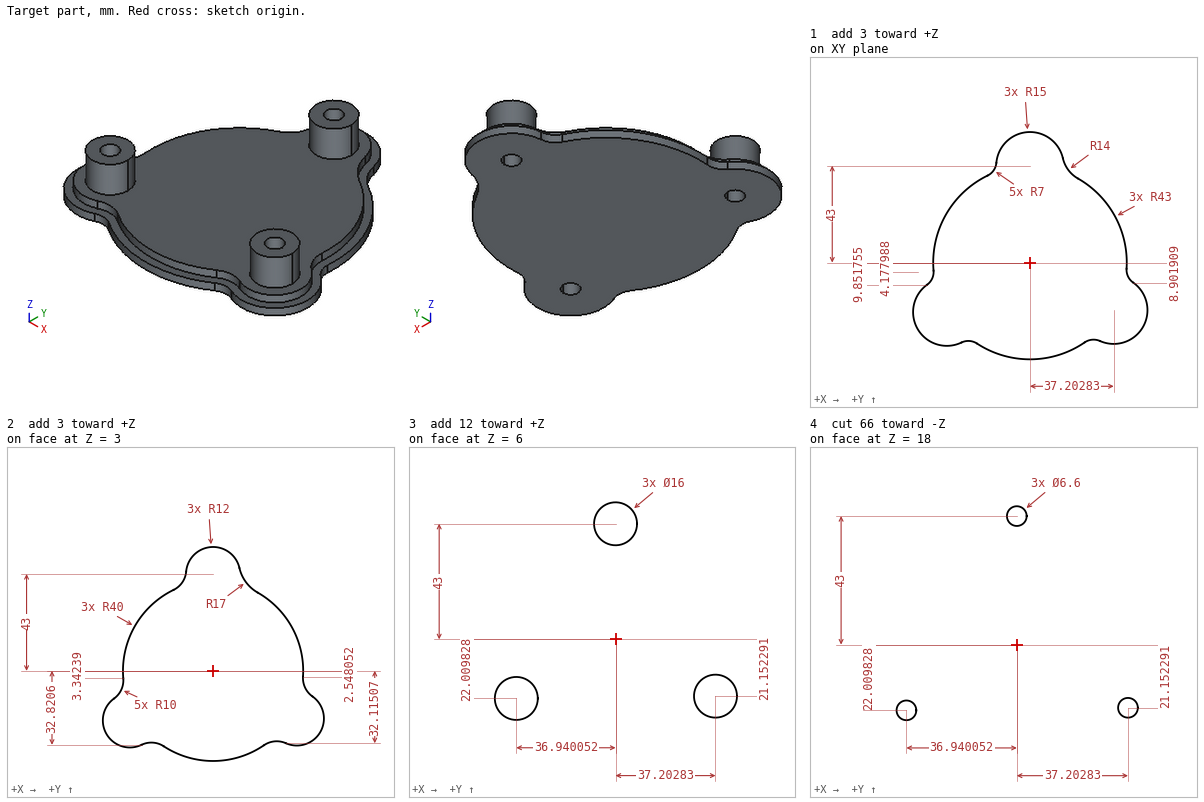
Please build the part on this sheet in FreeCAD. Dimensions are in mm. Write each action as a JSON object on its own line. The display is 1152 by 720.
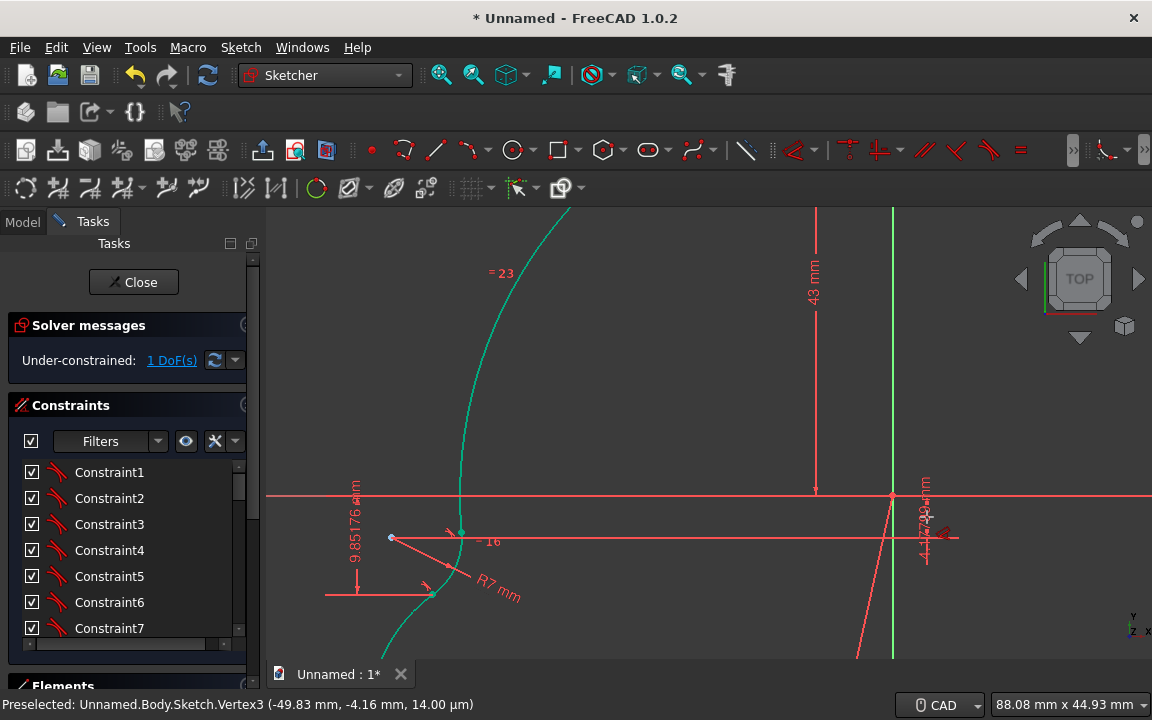
{"action": "scroll", "coordinate": [531, 438], "scroll_direction": "down", "scroll_amount": 6}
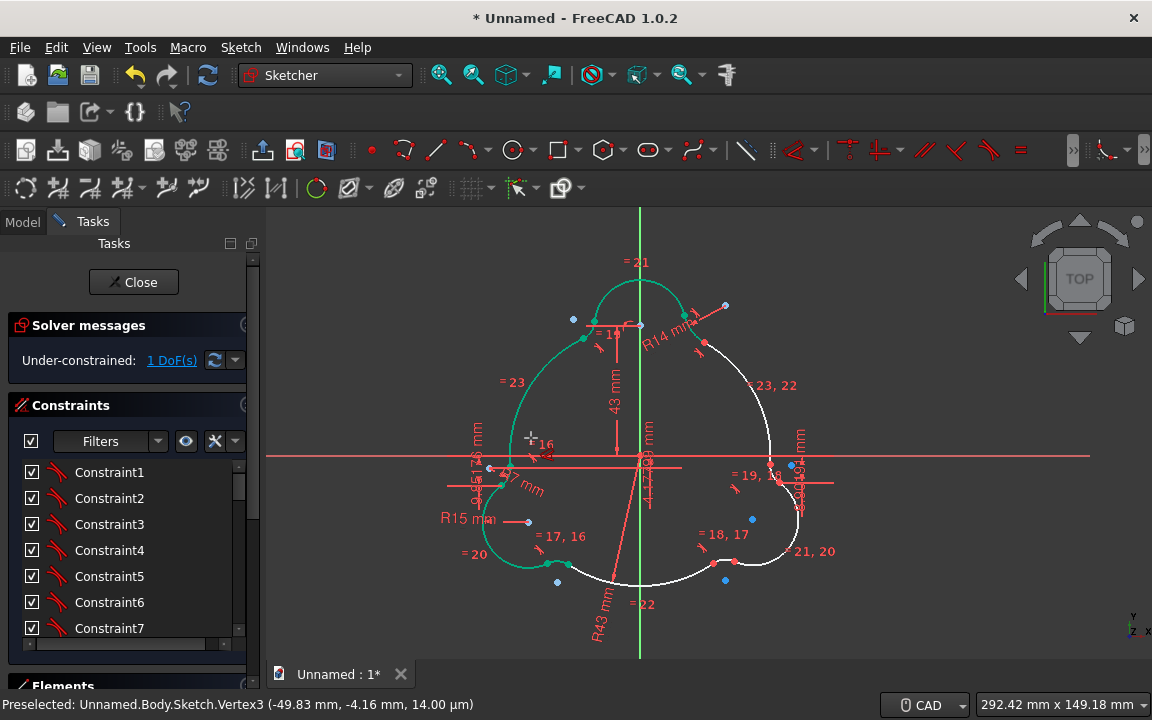
{"action": "left_click", "coordinate": [753, 520]}
{"action": "left_click", "coordinate": [697, 554]}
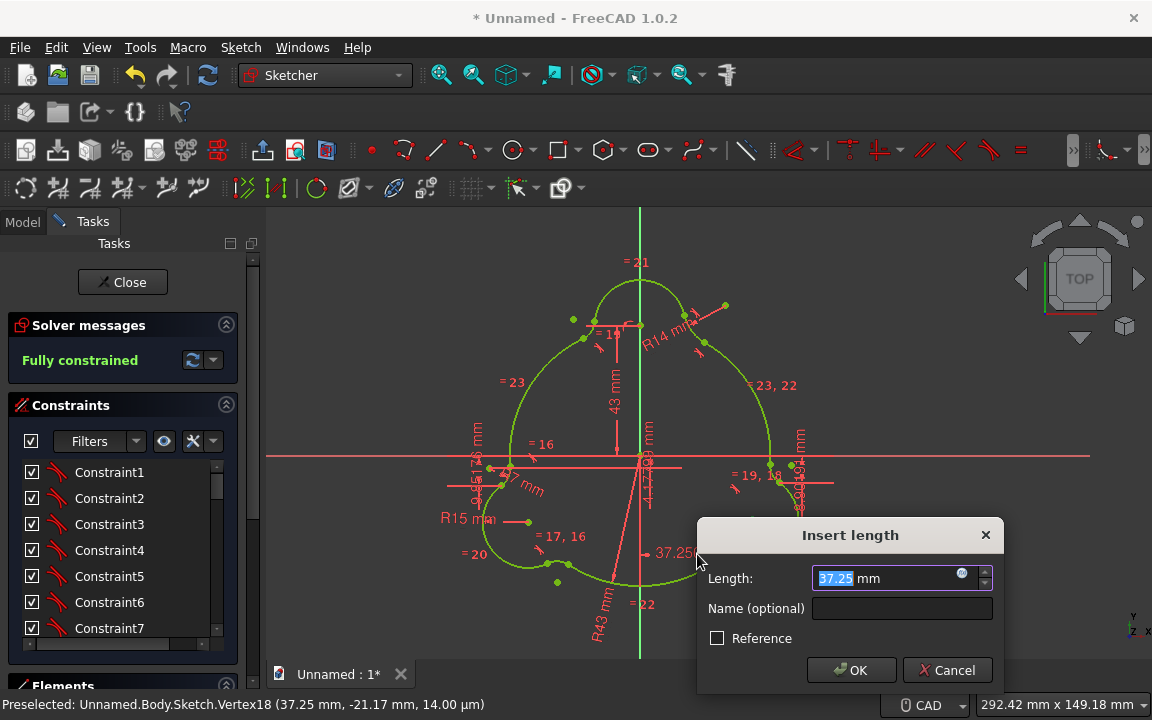
{"action": "type", "text": "37.20283"}
{"action": "key", "text": "Return"}
{"action": "key", "text": "Escape"}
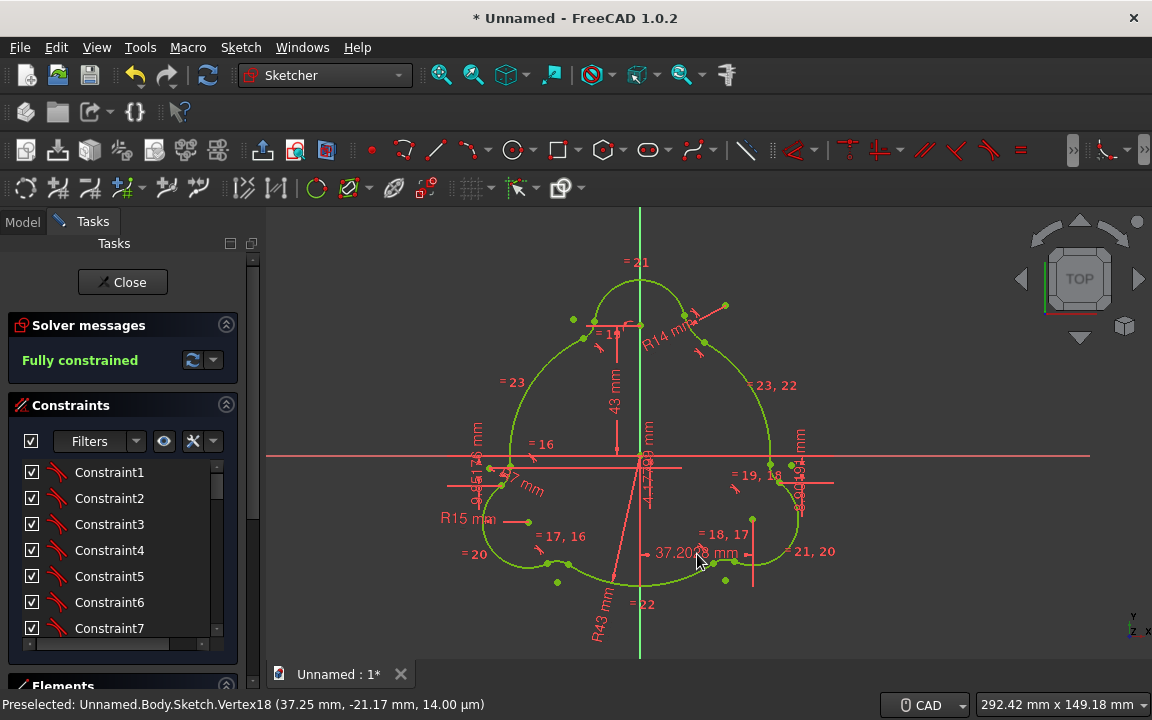
{"action": "left_click", "coordinate": [123, 282]}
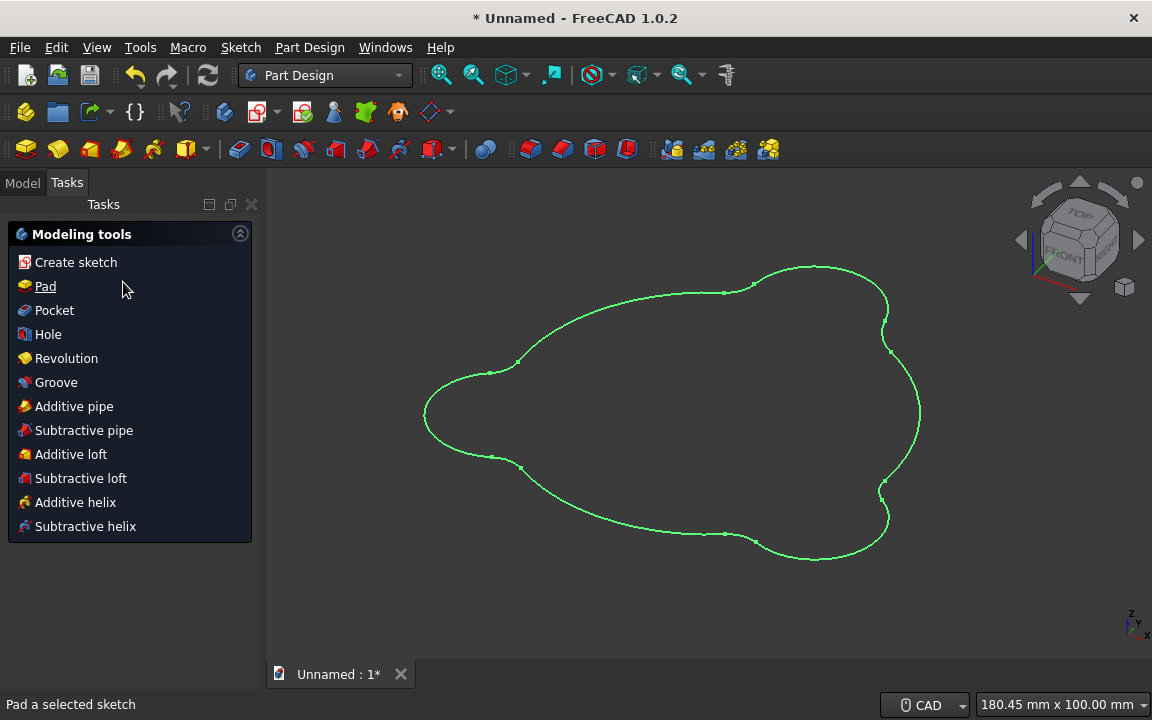
{"action": "left_click", "coordinate": [26, 150]}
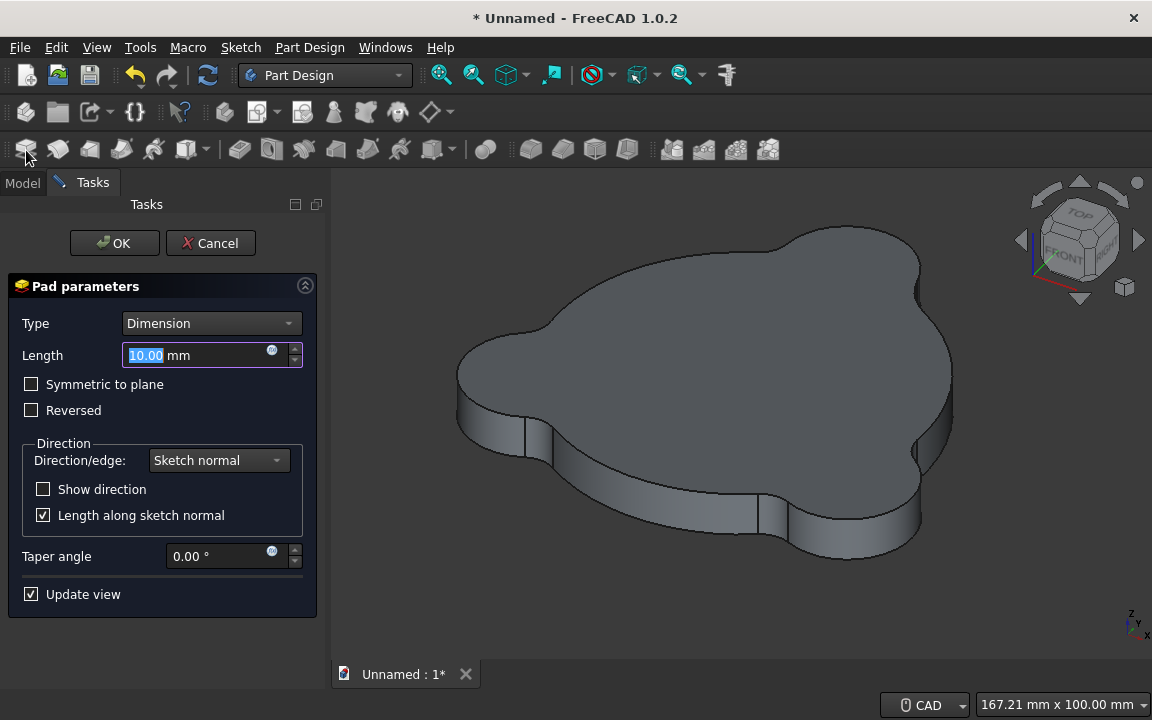
{"action": "type", "text": "3"}
{"action": "key", "text": "Tab"}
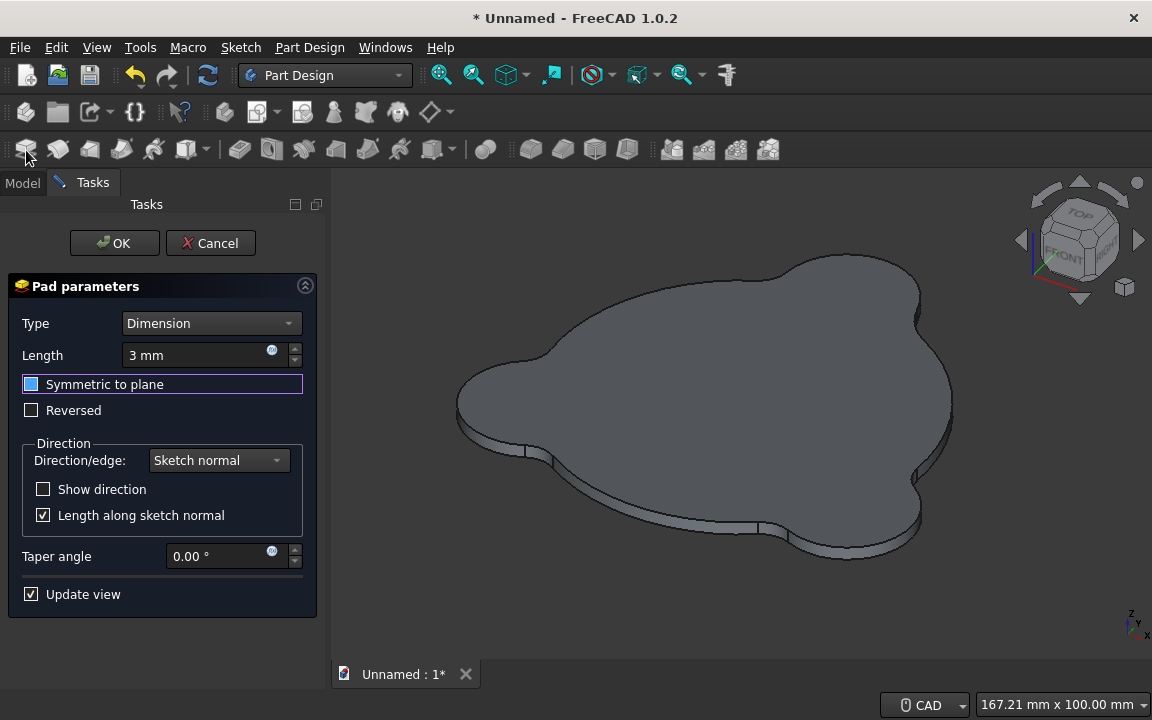
{"action": "left_click", "coordinate": [115, 243]}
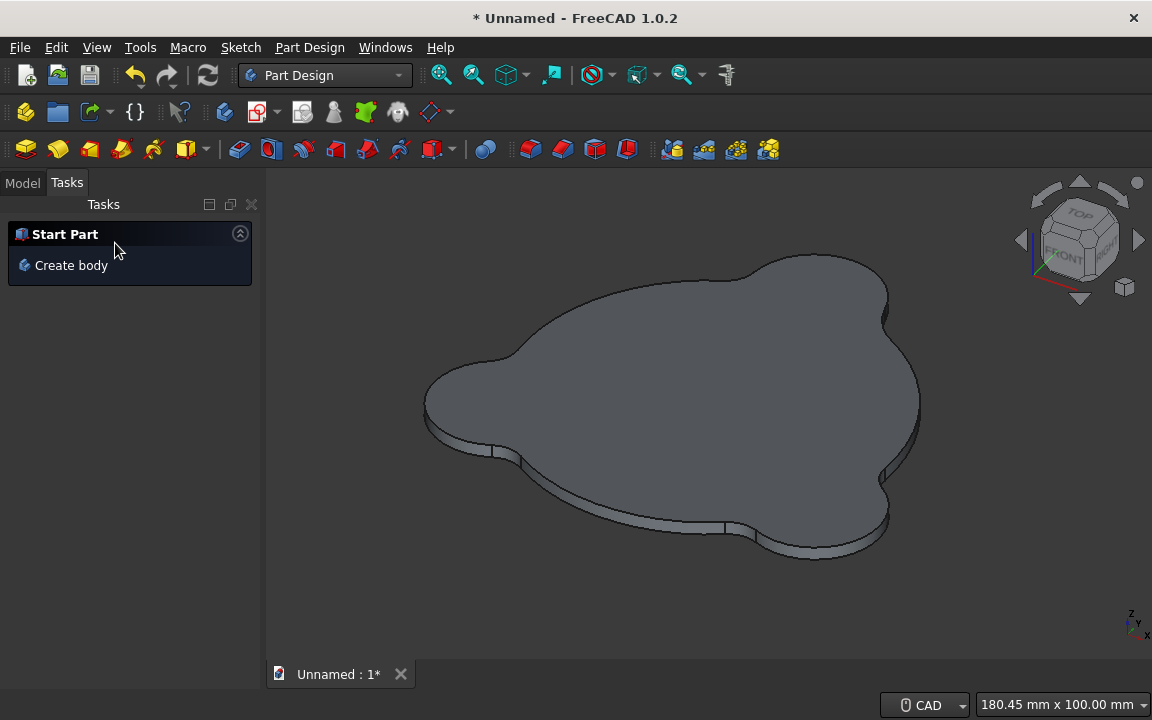
{"action": "left_click", "coordinate": [728, 382]}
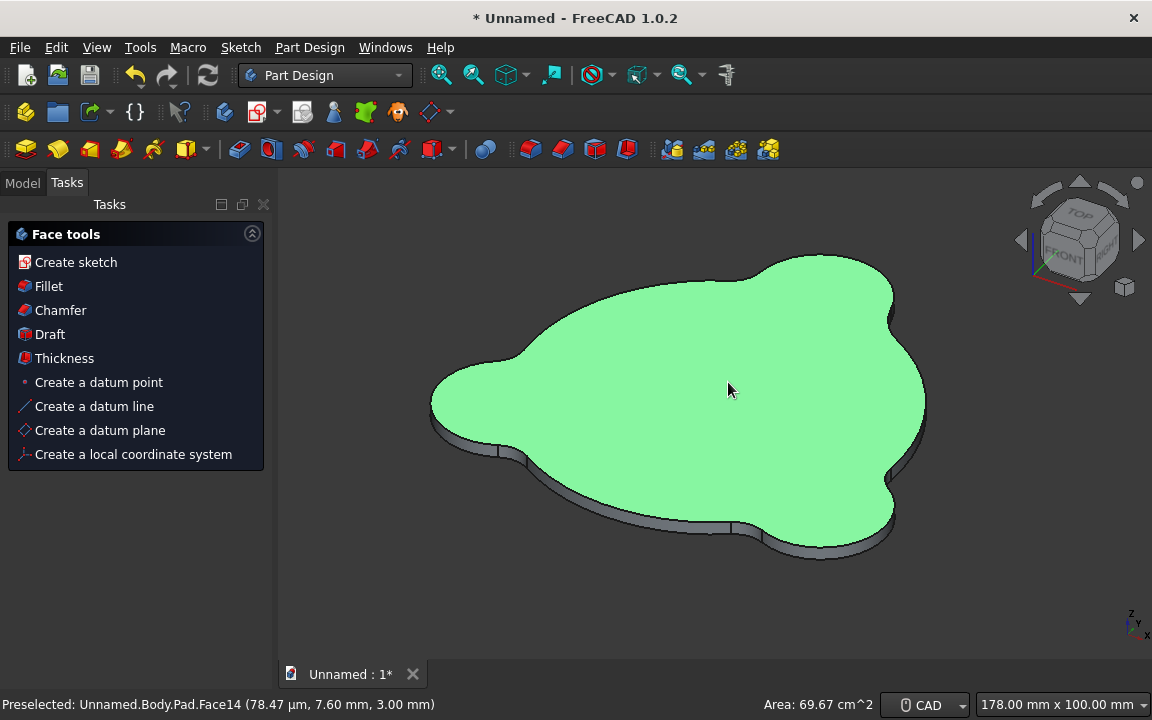
{"action": "left_click", "coordinate": [258, 112]}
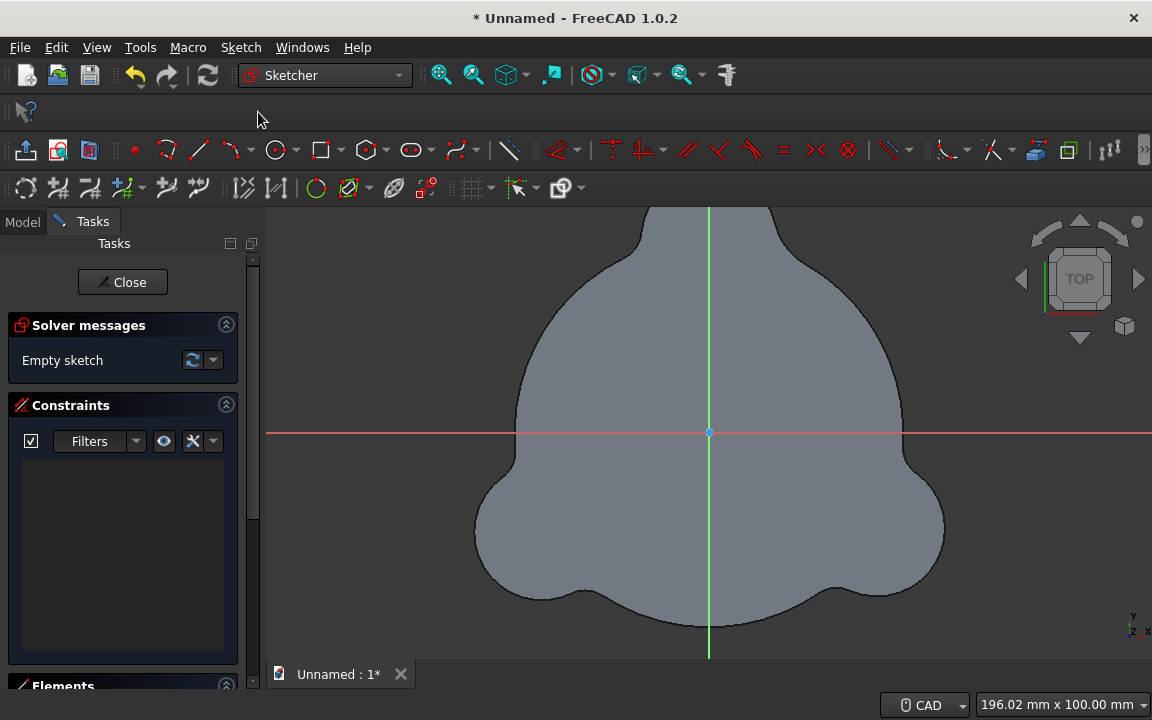
{"action": "scroll", "coordinate": [499, 502], "scroll_direction": "down", "scroll_amount": 2}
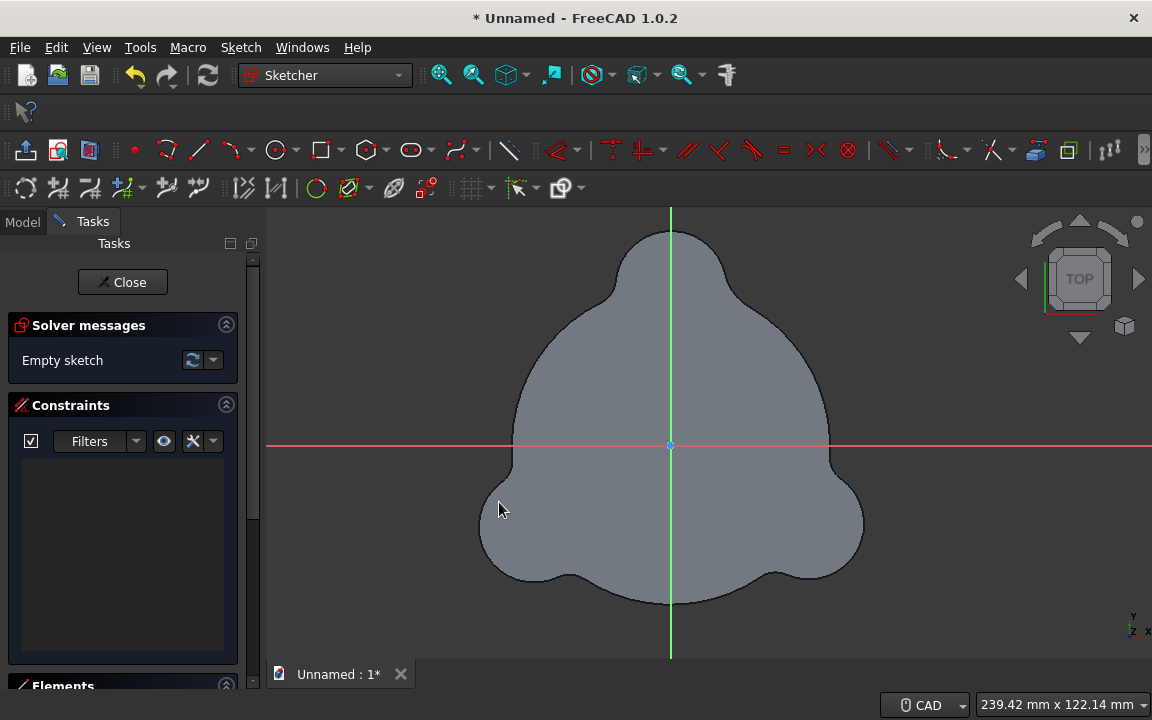
{"action": "key", "text": "g 3 a"}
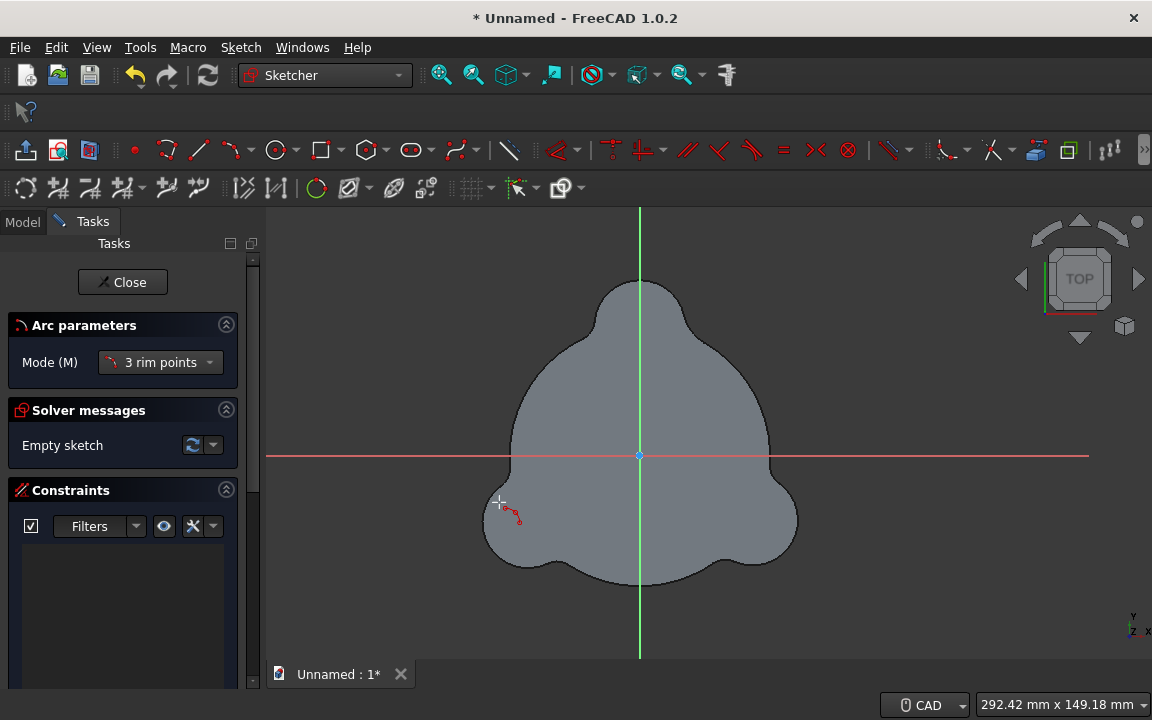
{"action": "left_click", "coordinate": [700, 351]}
{"action": "left_click", "coordinate": [675, 318]}